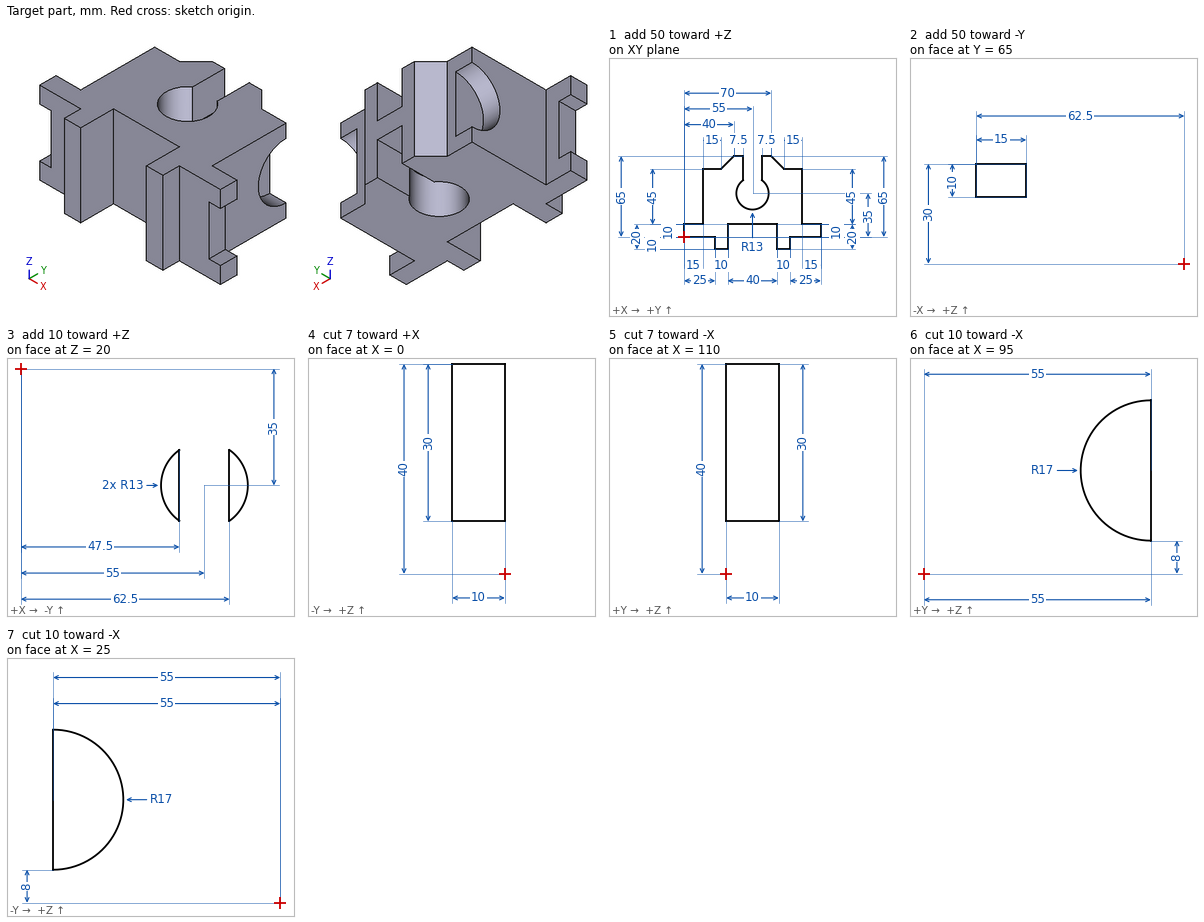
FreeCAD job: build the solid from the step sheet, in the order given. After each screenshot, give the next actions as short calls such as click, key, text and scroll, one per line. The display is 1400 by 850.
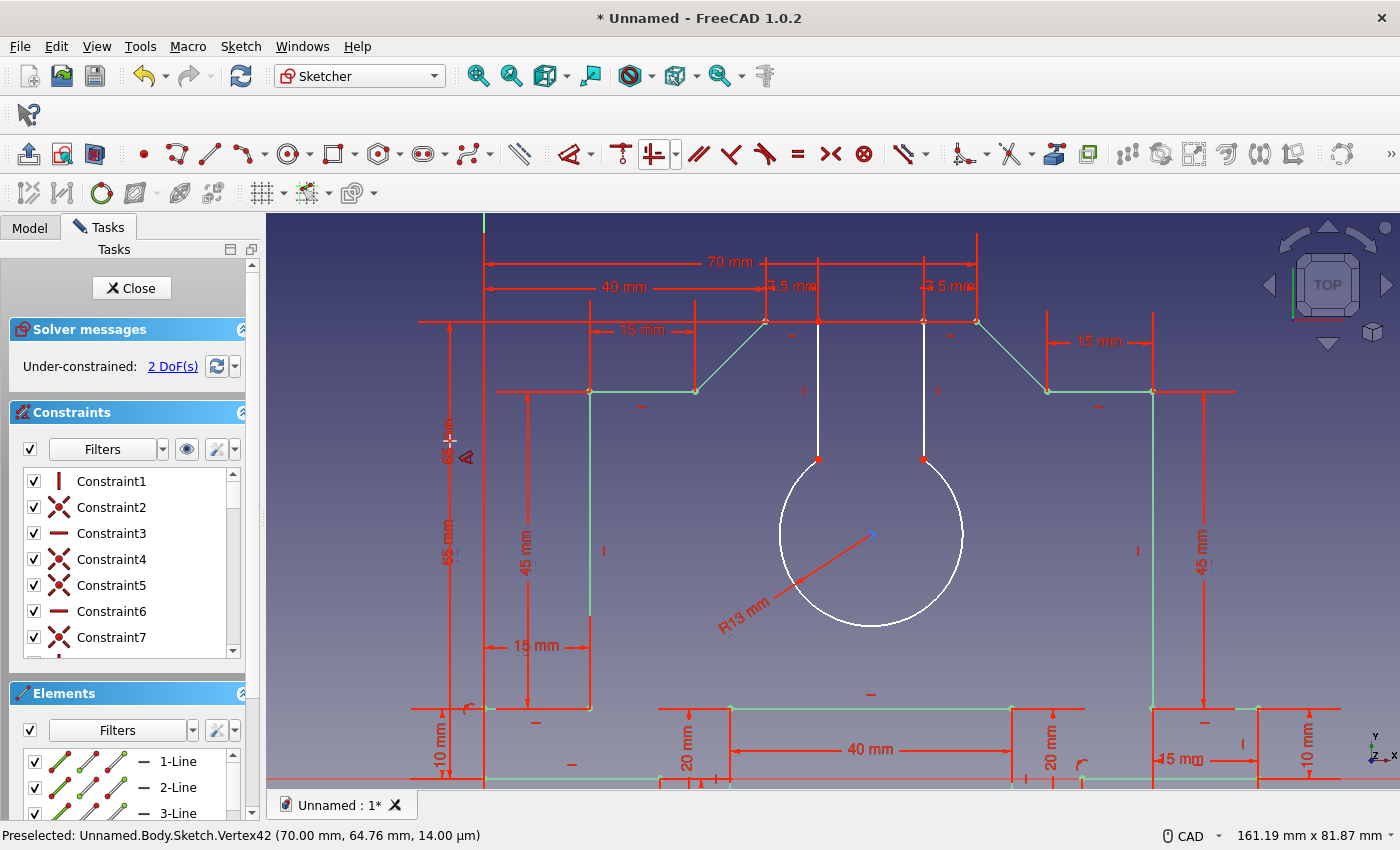
click(871, 535)
click(678, 501)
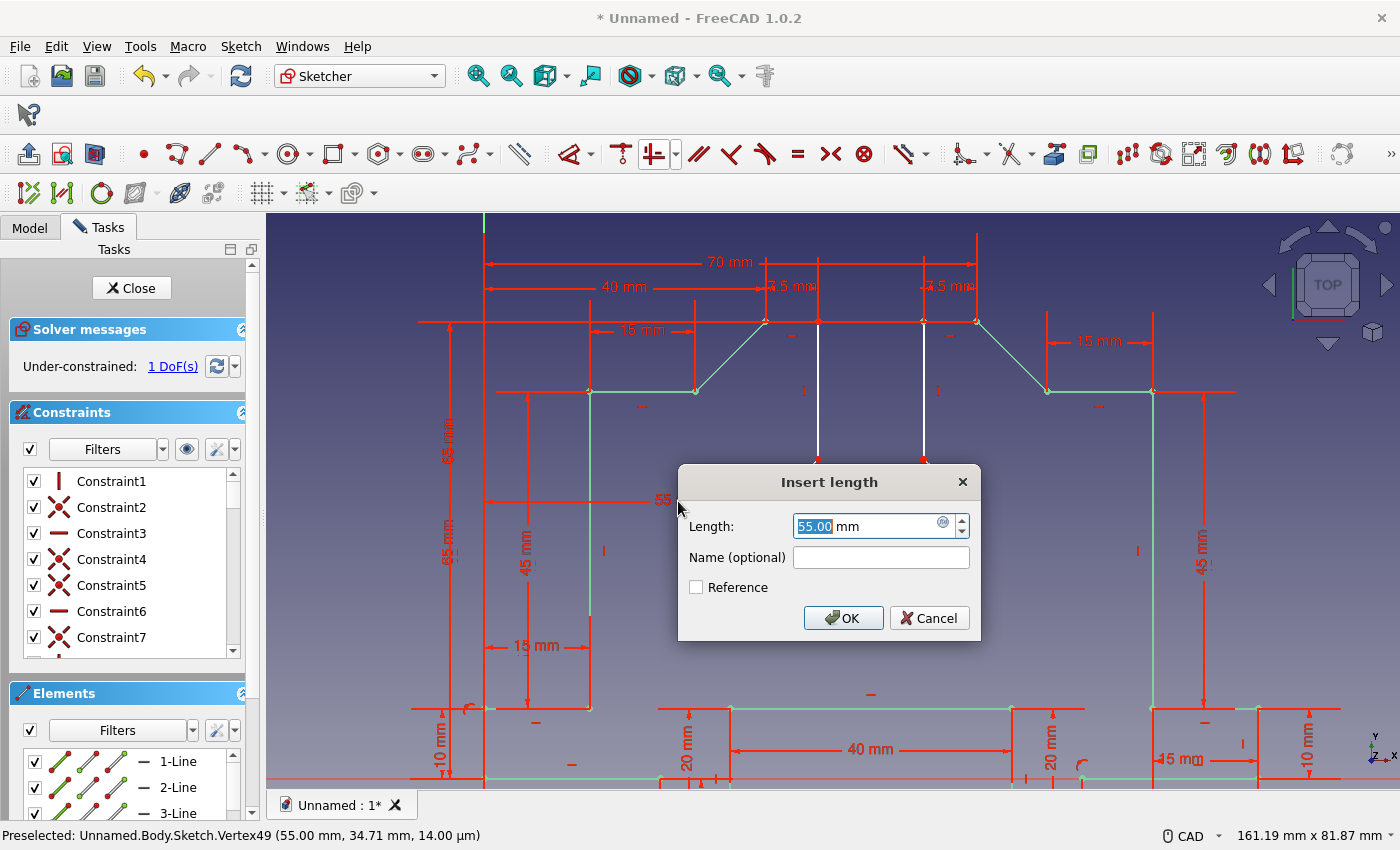
text(55)
key(Return)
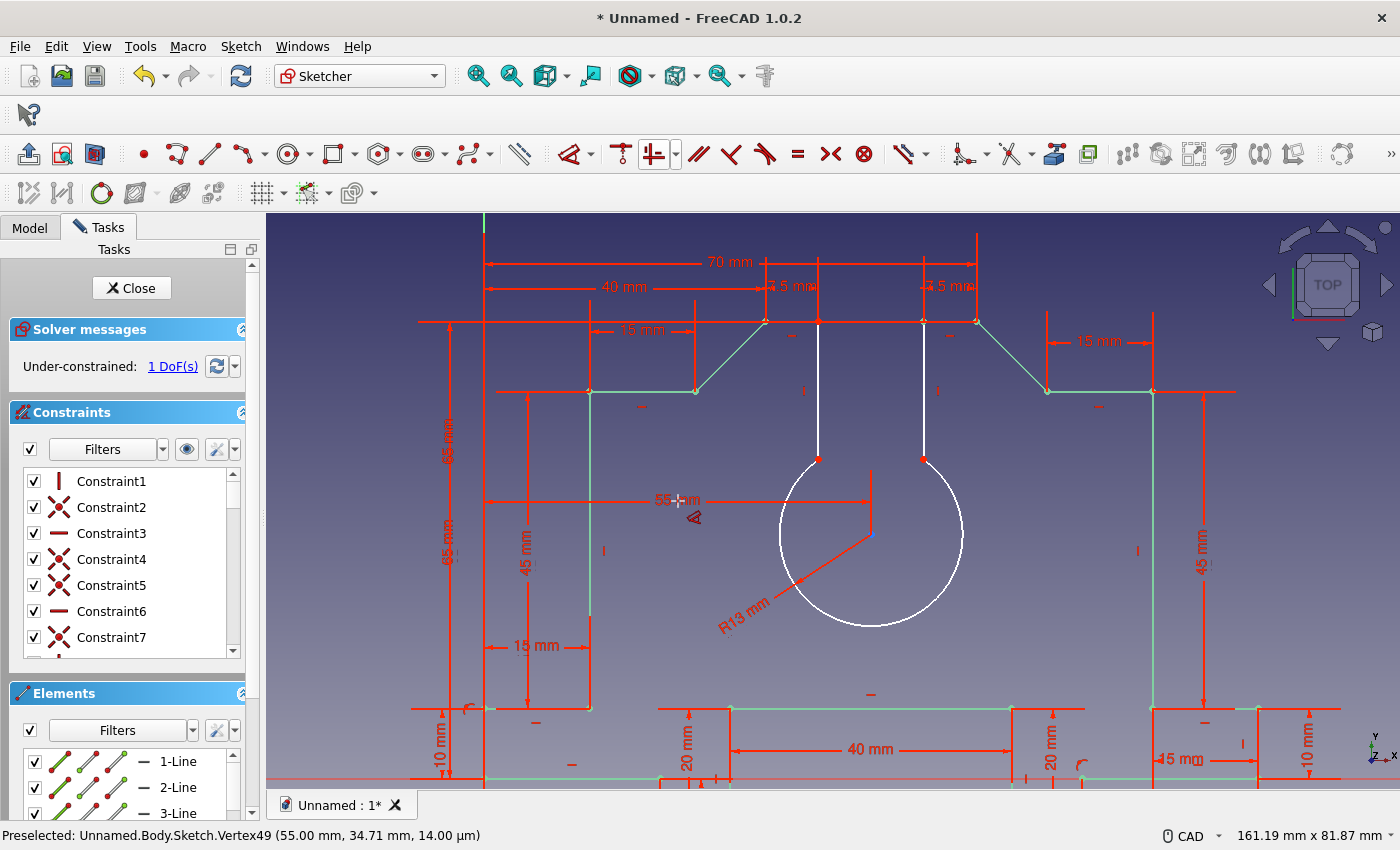
click(871, 535)
click(450, 648)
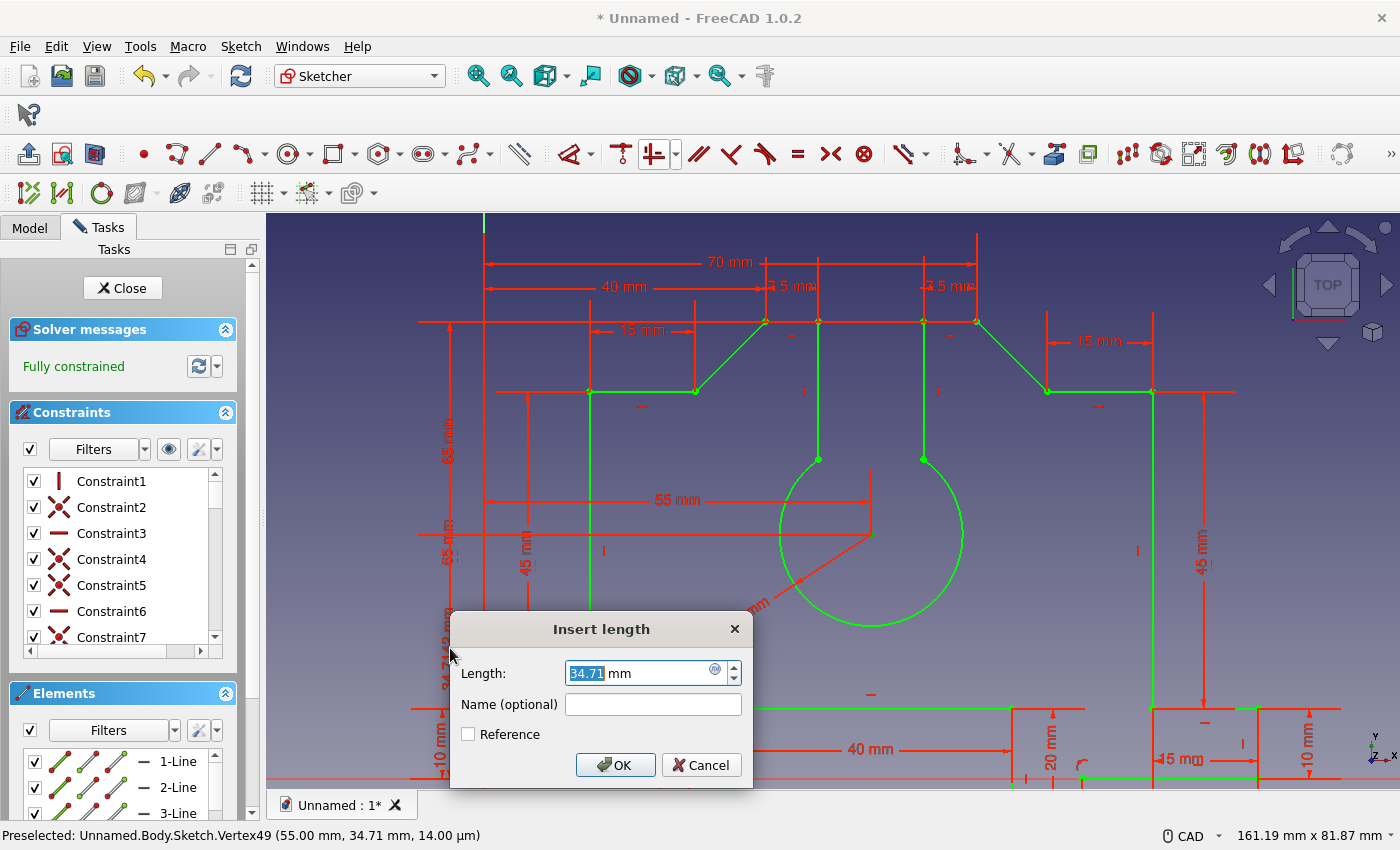
text(35)
key(Return)
key(Escape)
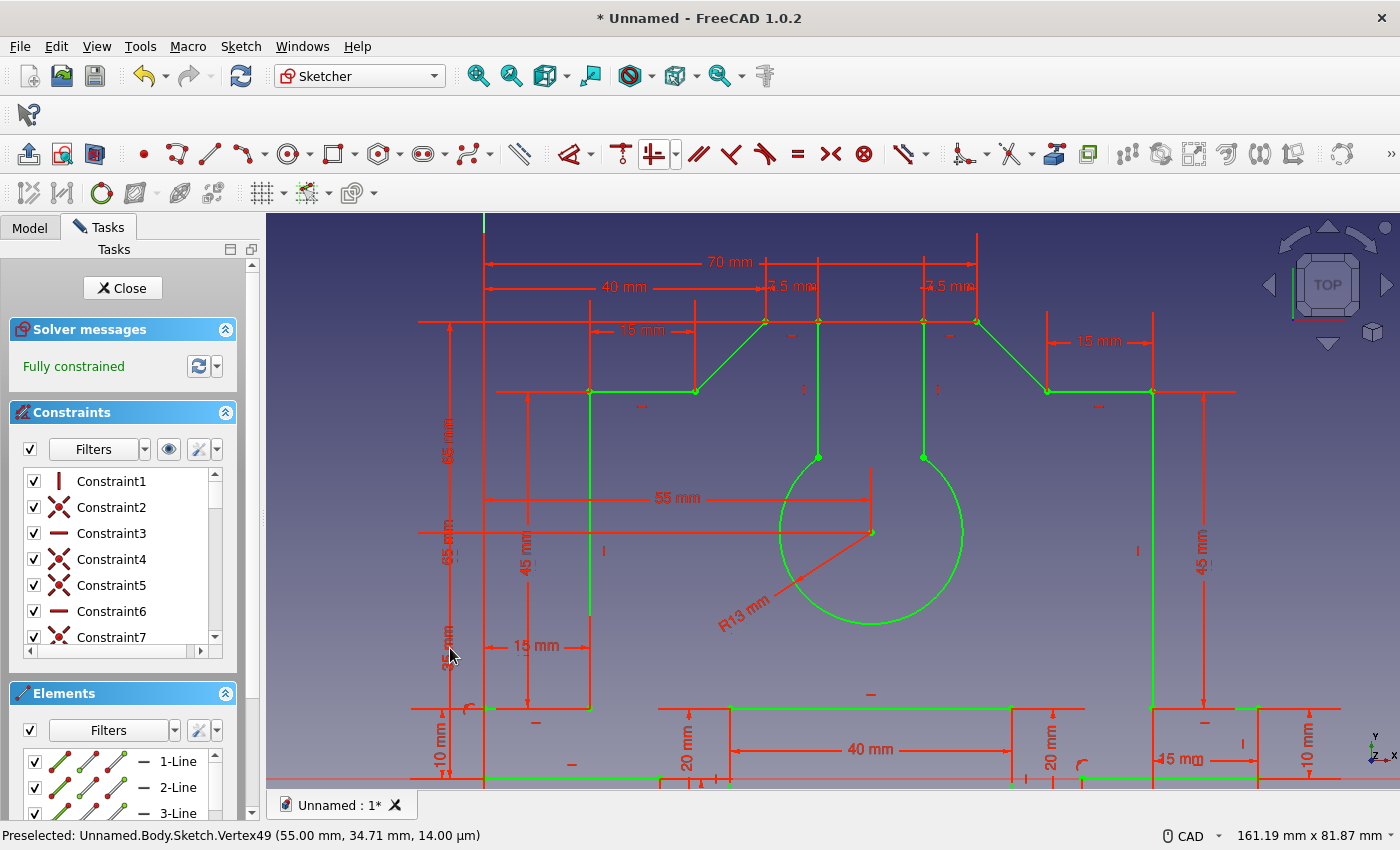
click(123, 288)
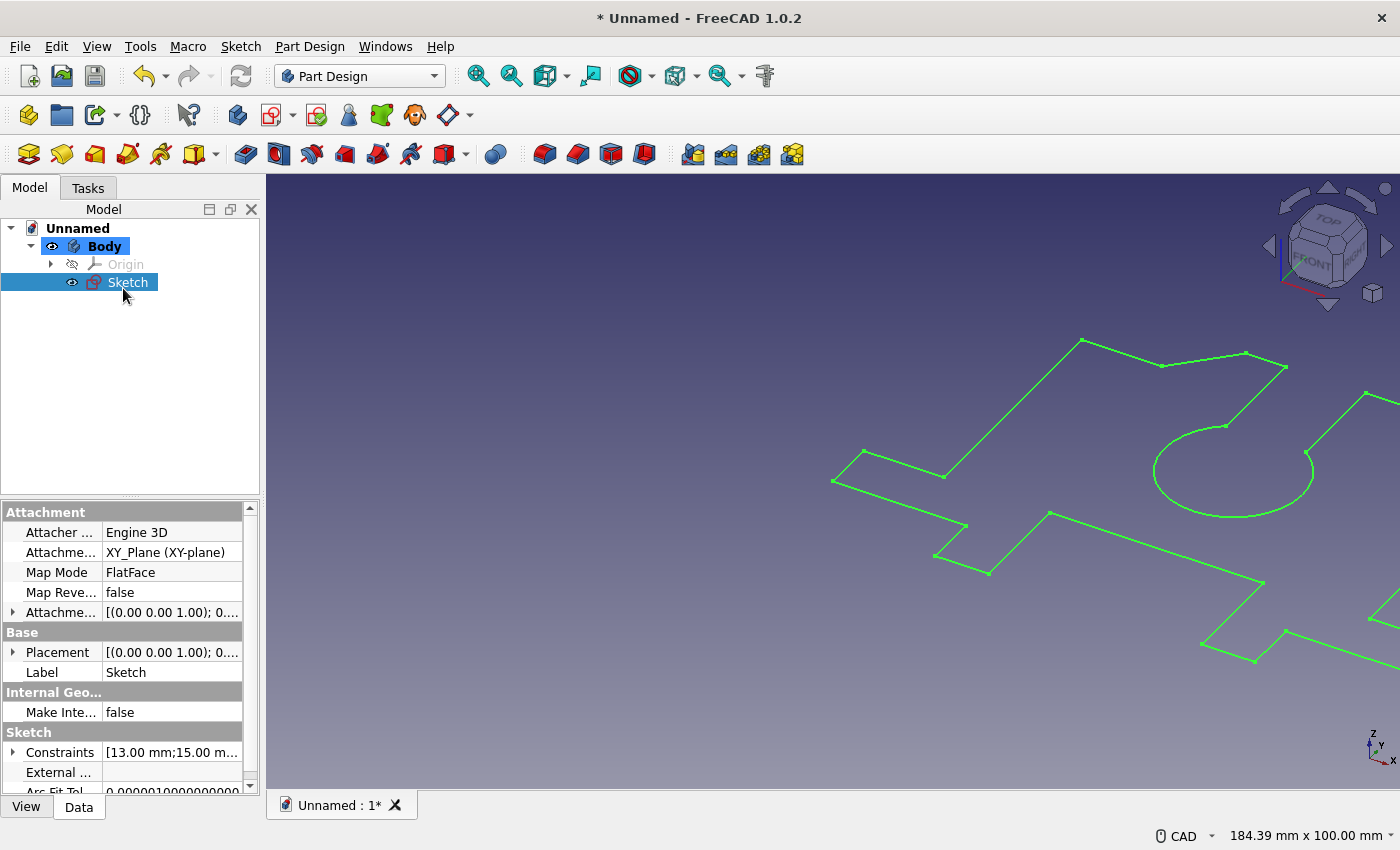
click(29, 154)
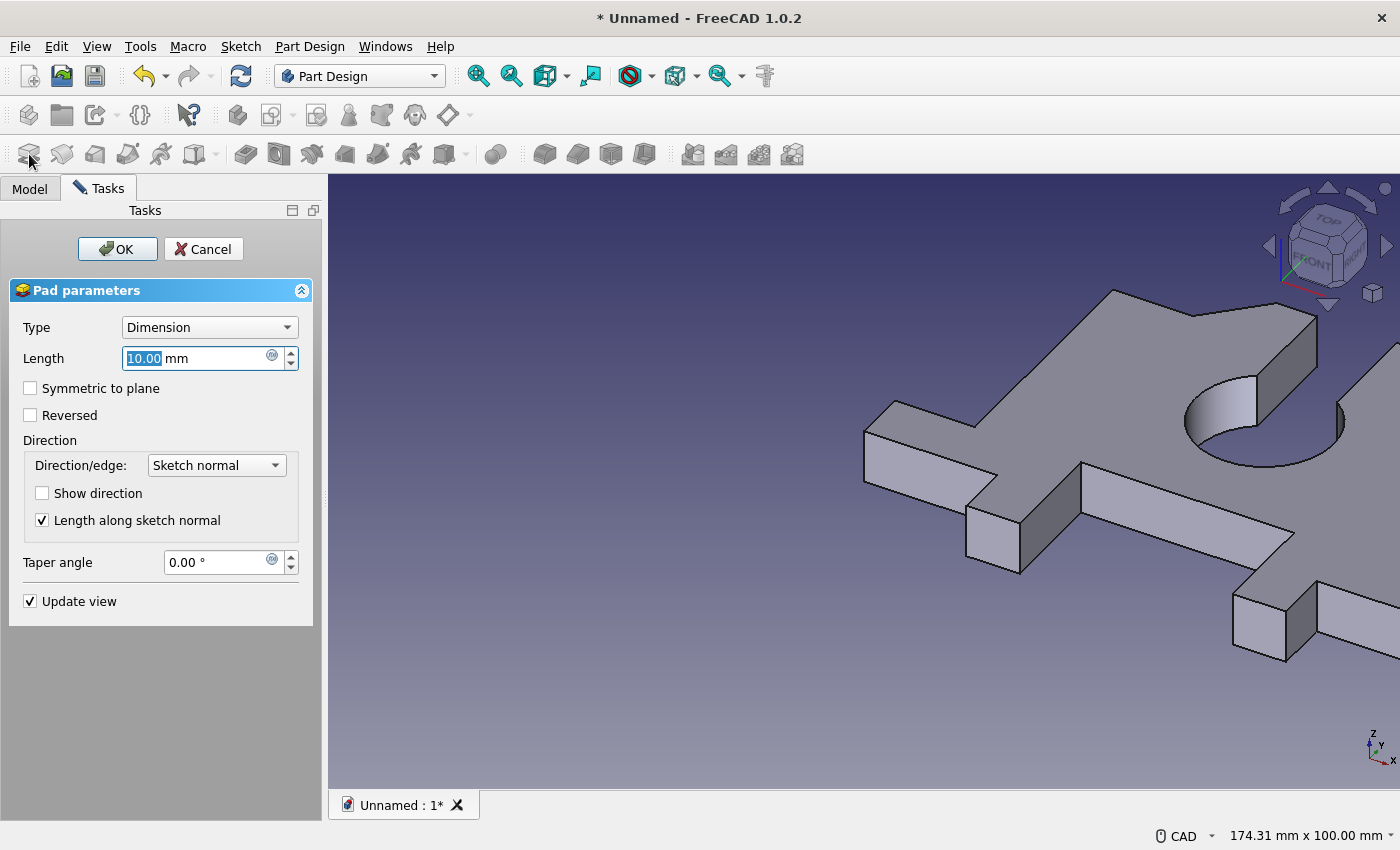
text(50)
key(Tab)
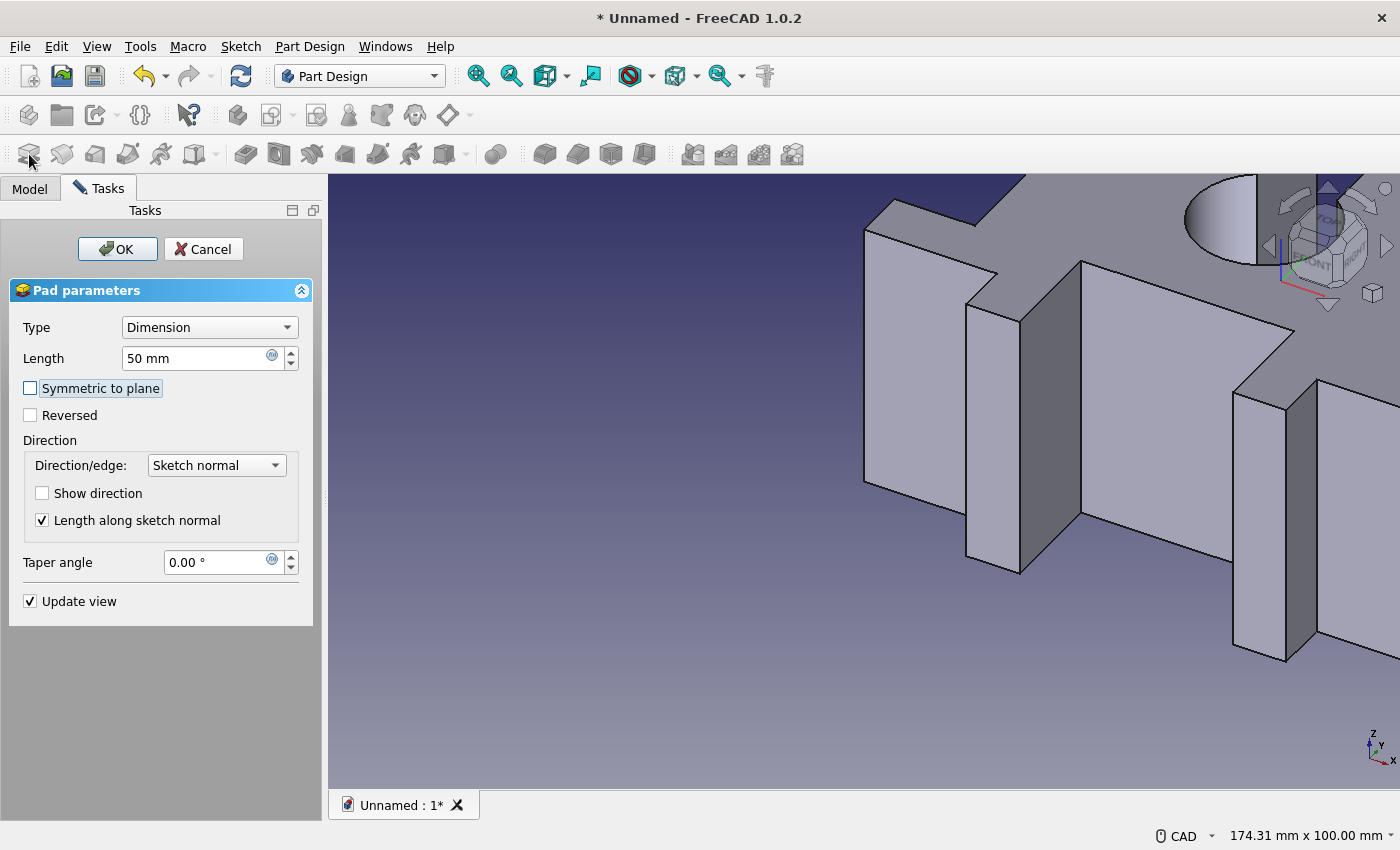
click(118, 249)